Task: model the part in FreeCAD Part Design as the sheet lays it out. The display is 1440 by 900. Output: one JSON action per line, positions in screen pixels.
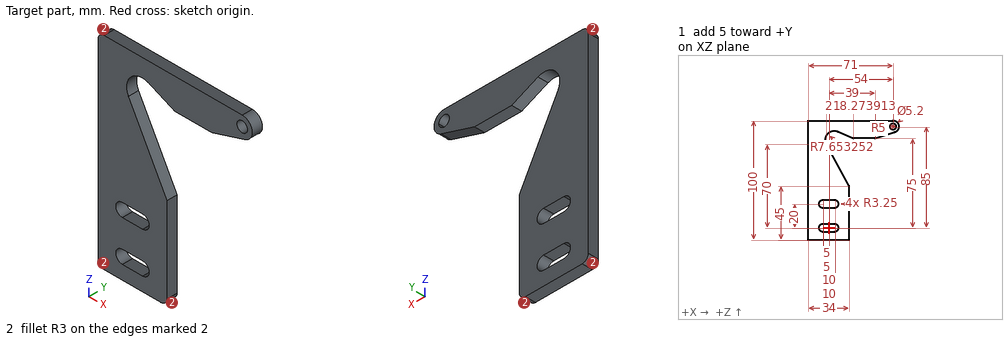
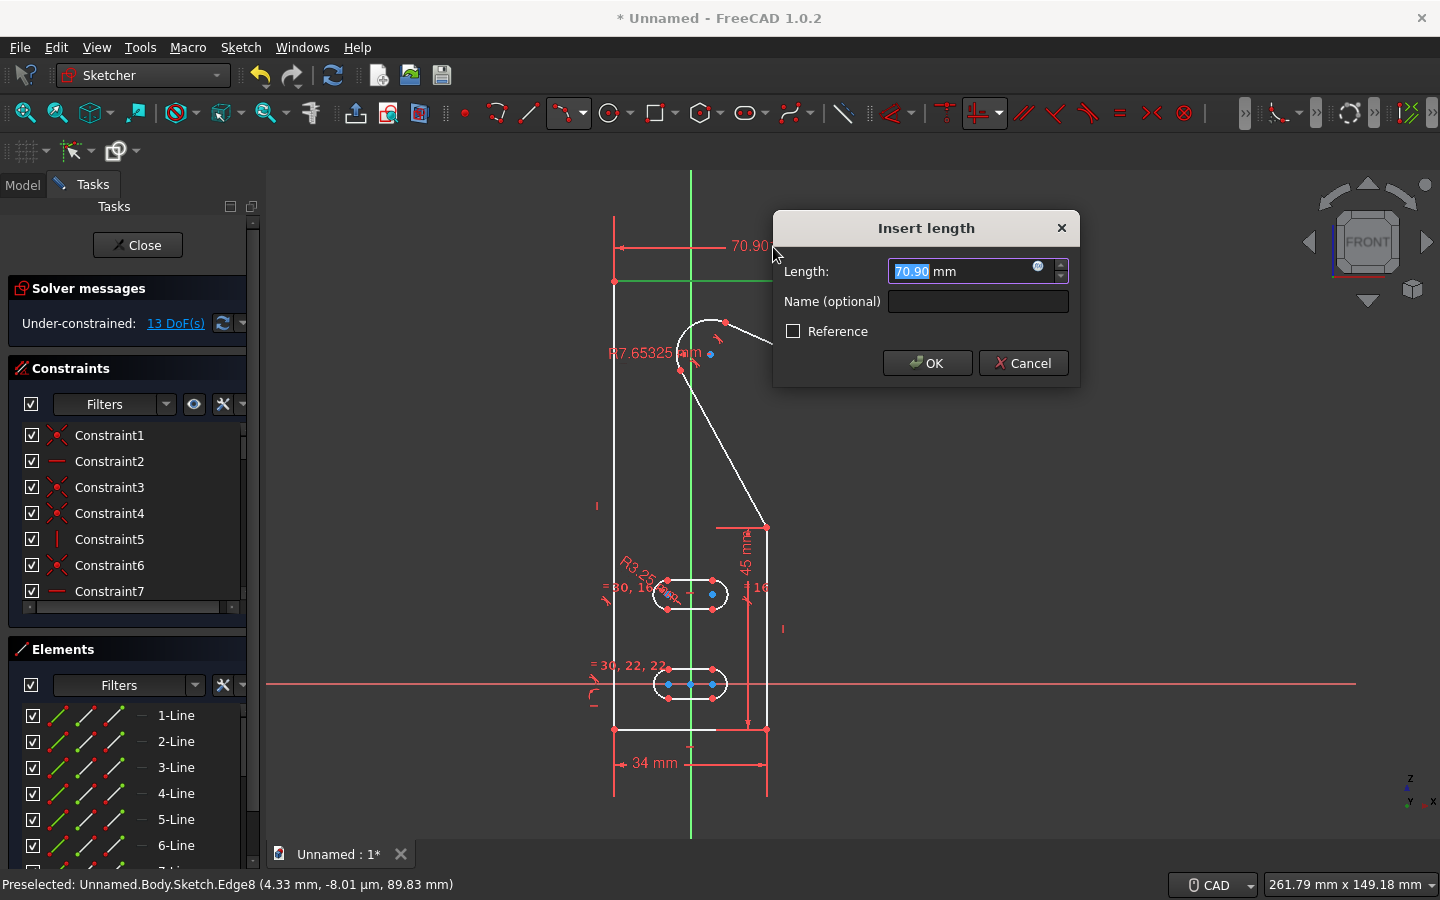
{"action": "type", "text": "71"}
{"action": "key", "text": "Return"}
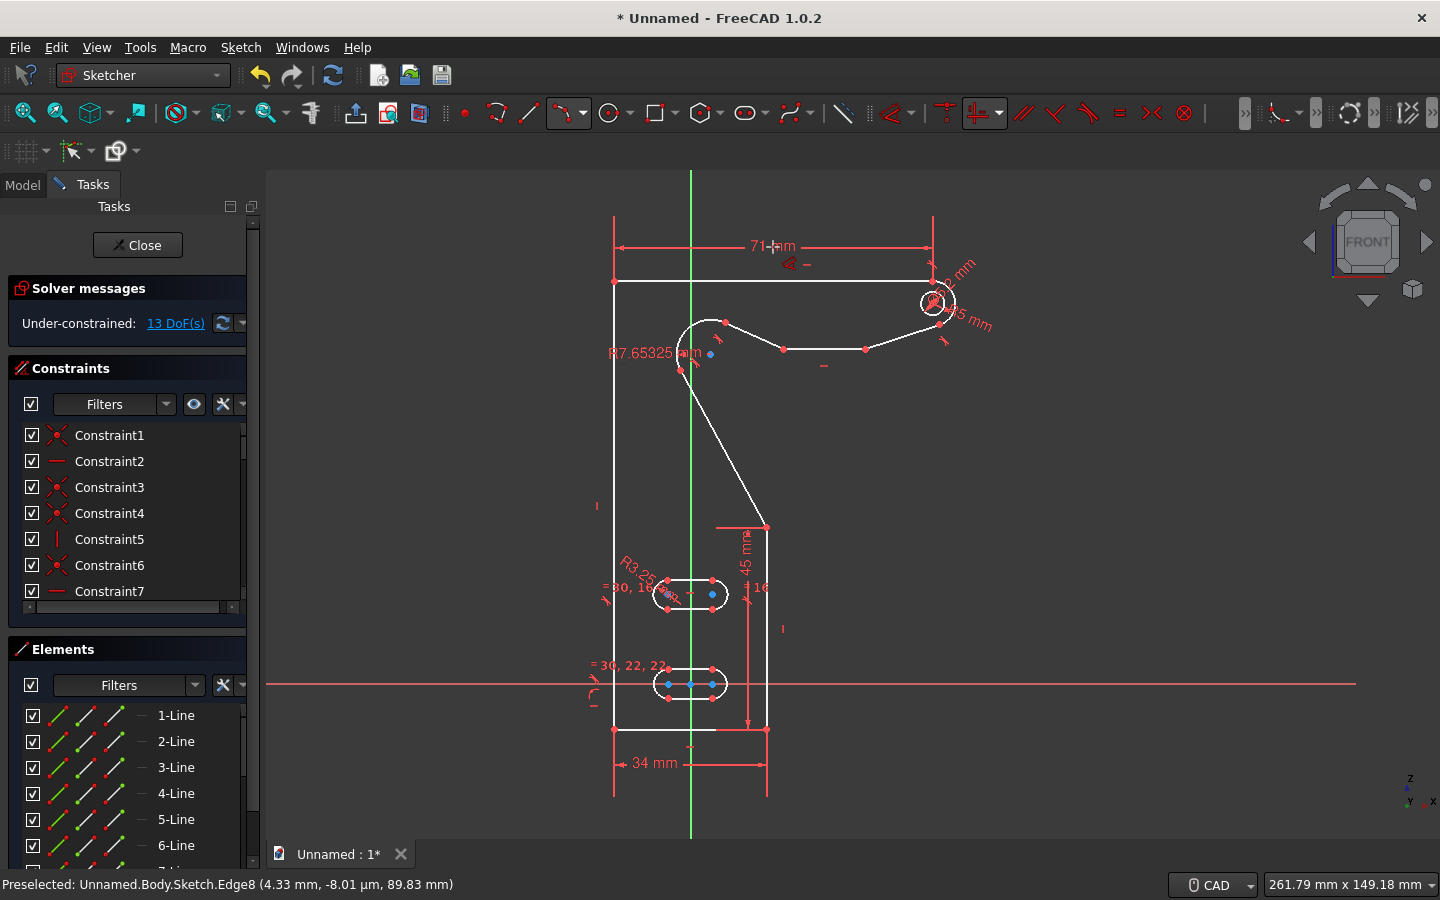
{"action": "scroll", "coordinate": [681, 580], "scroll_direction": "up", "scroll_amount": 3}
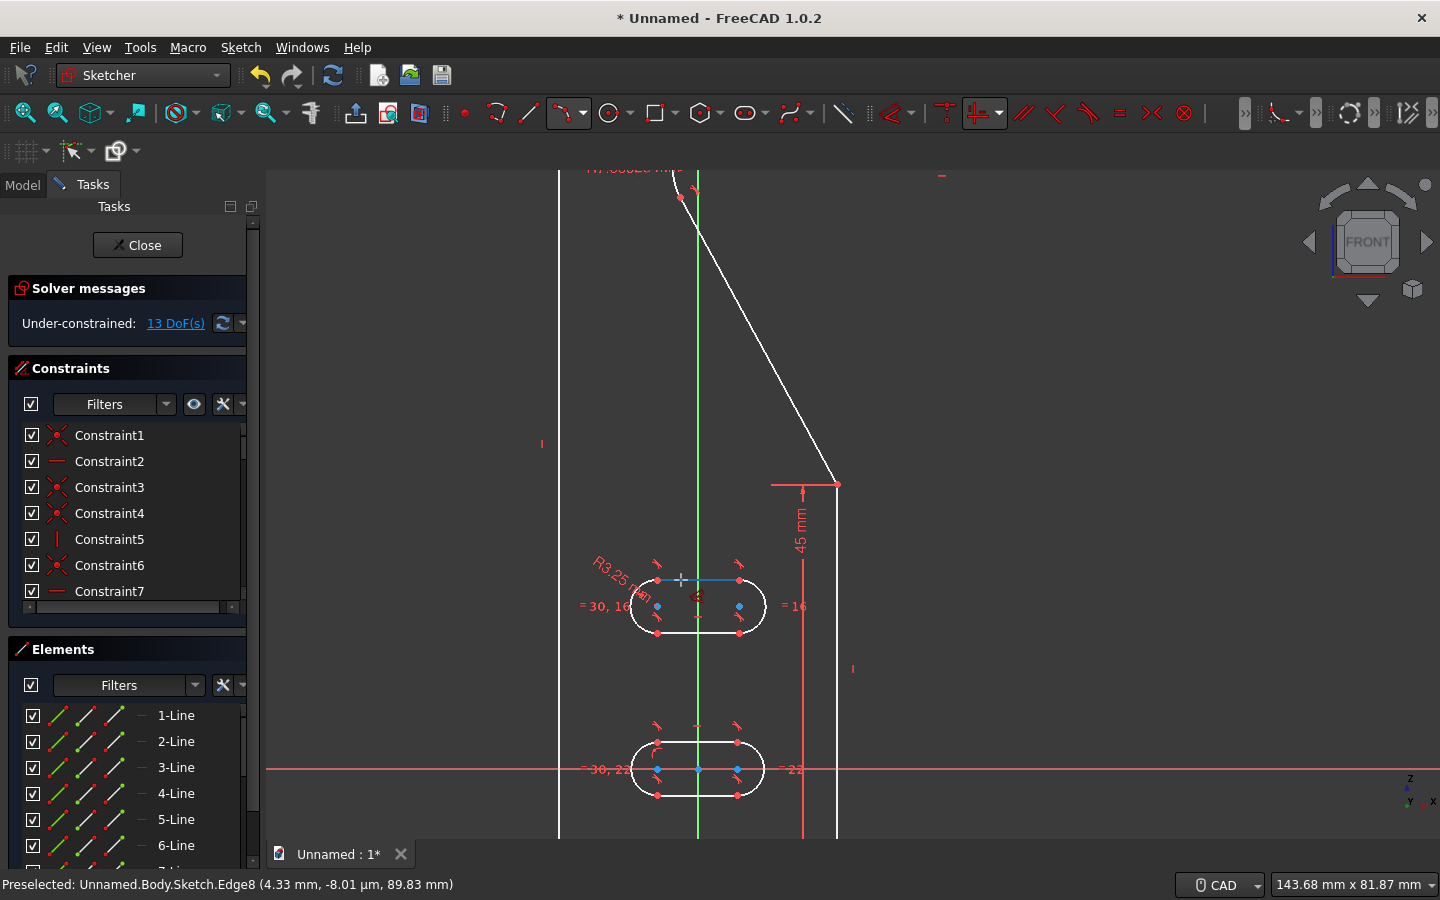
{"action": "left_click", "coordinate": [682, 580]}
{"action": "left_click", "coordinate": [679, 614]}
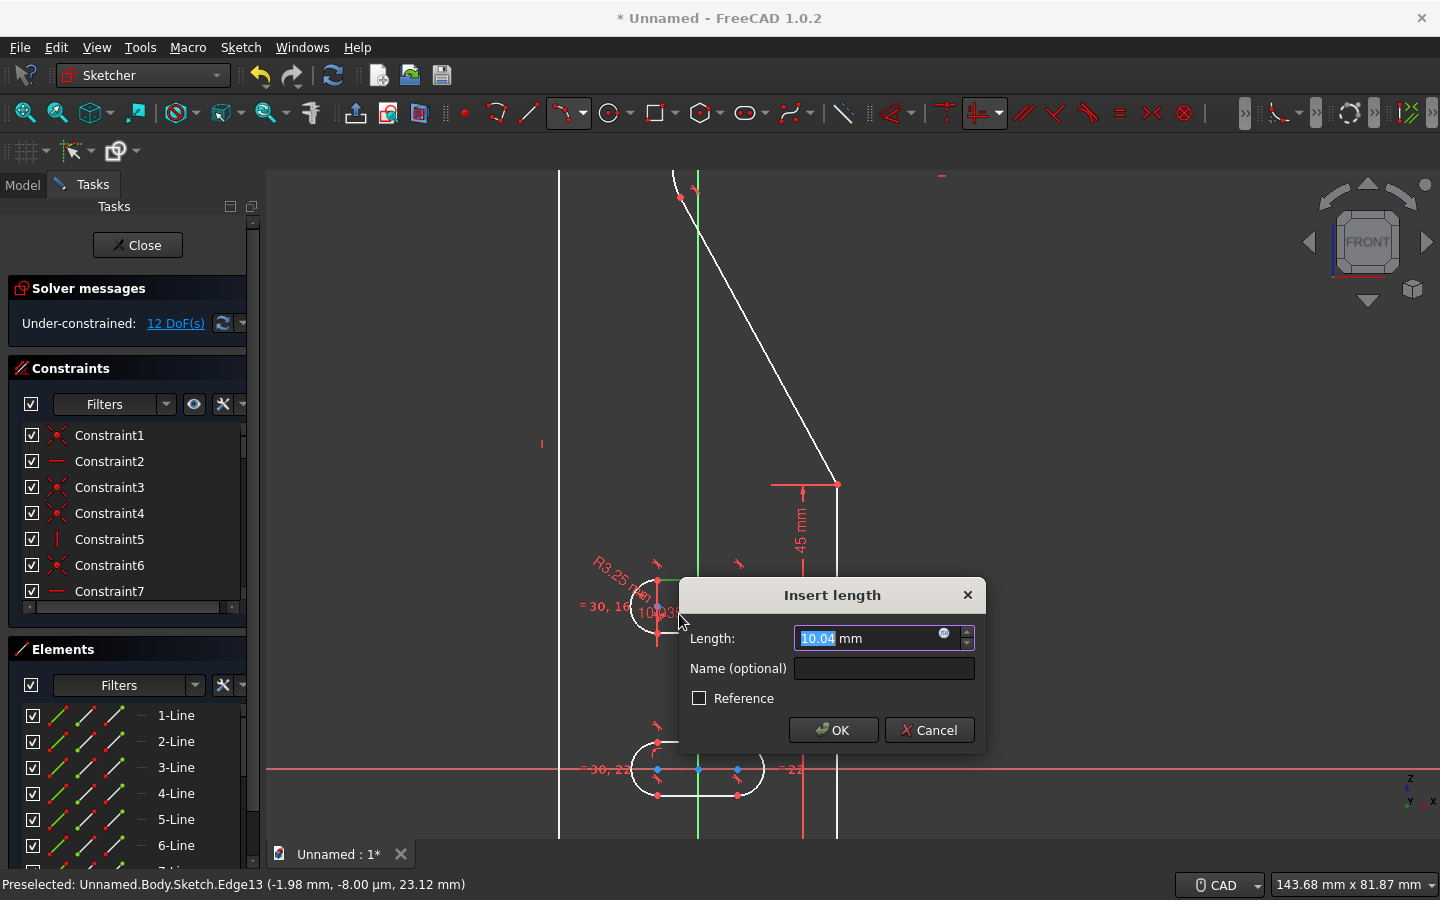
{"action": "type", "text": "10"}
{"action": "key", "text": "Return"}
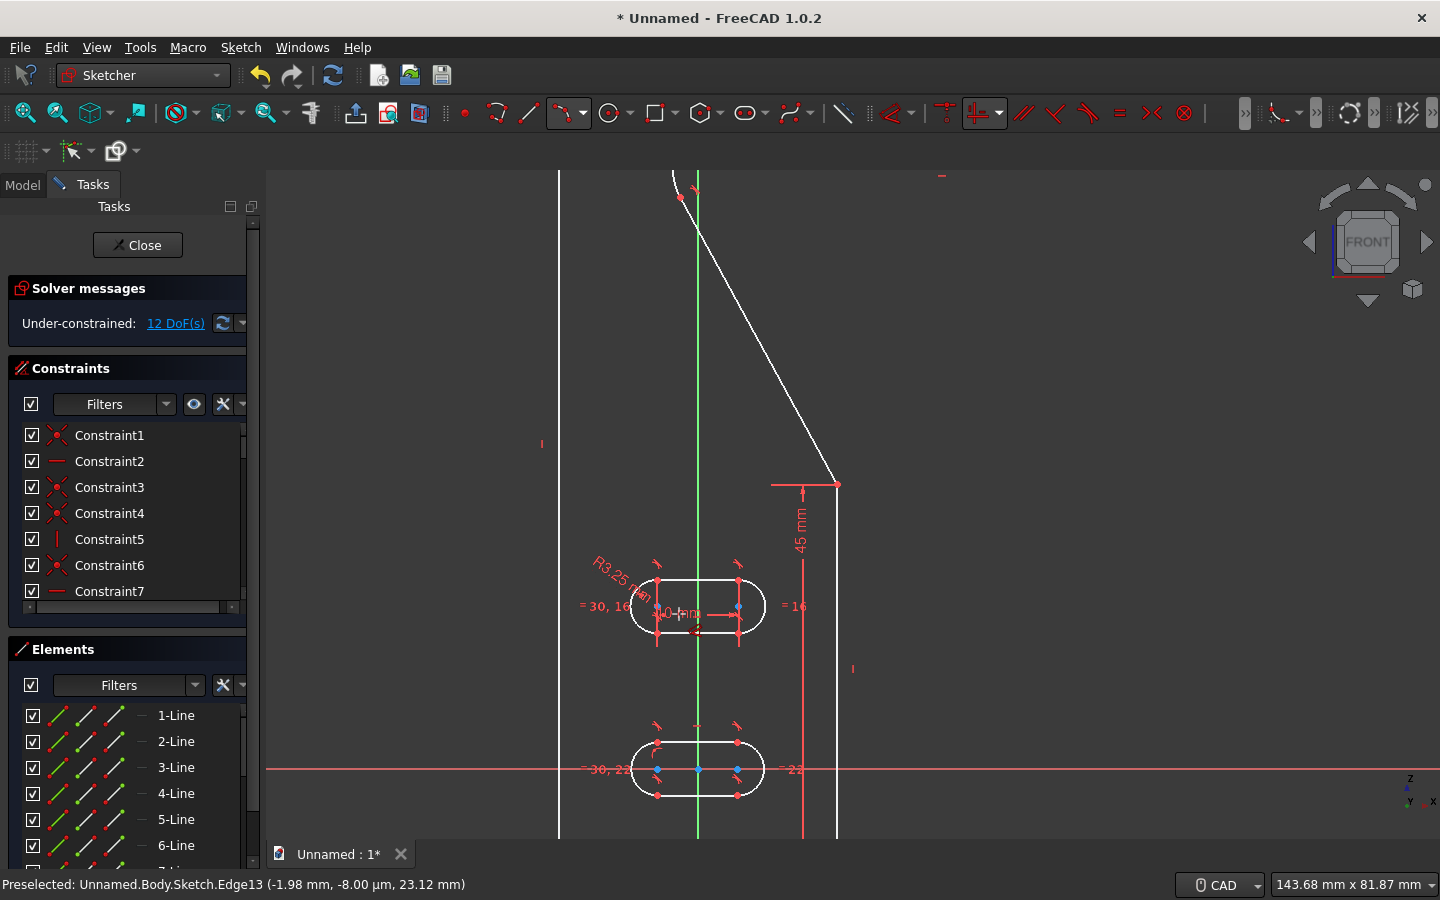
{"action": "left_click", "coordinate": [682, 742]}
{"action": "left_click", "coordinate": [679, 708]}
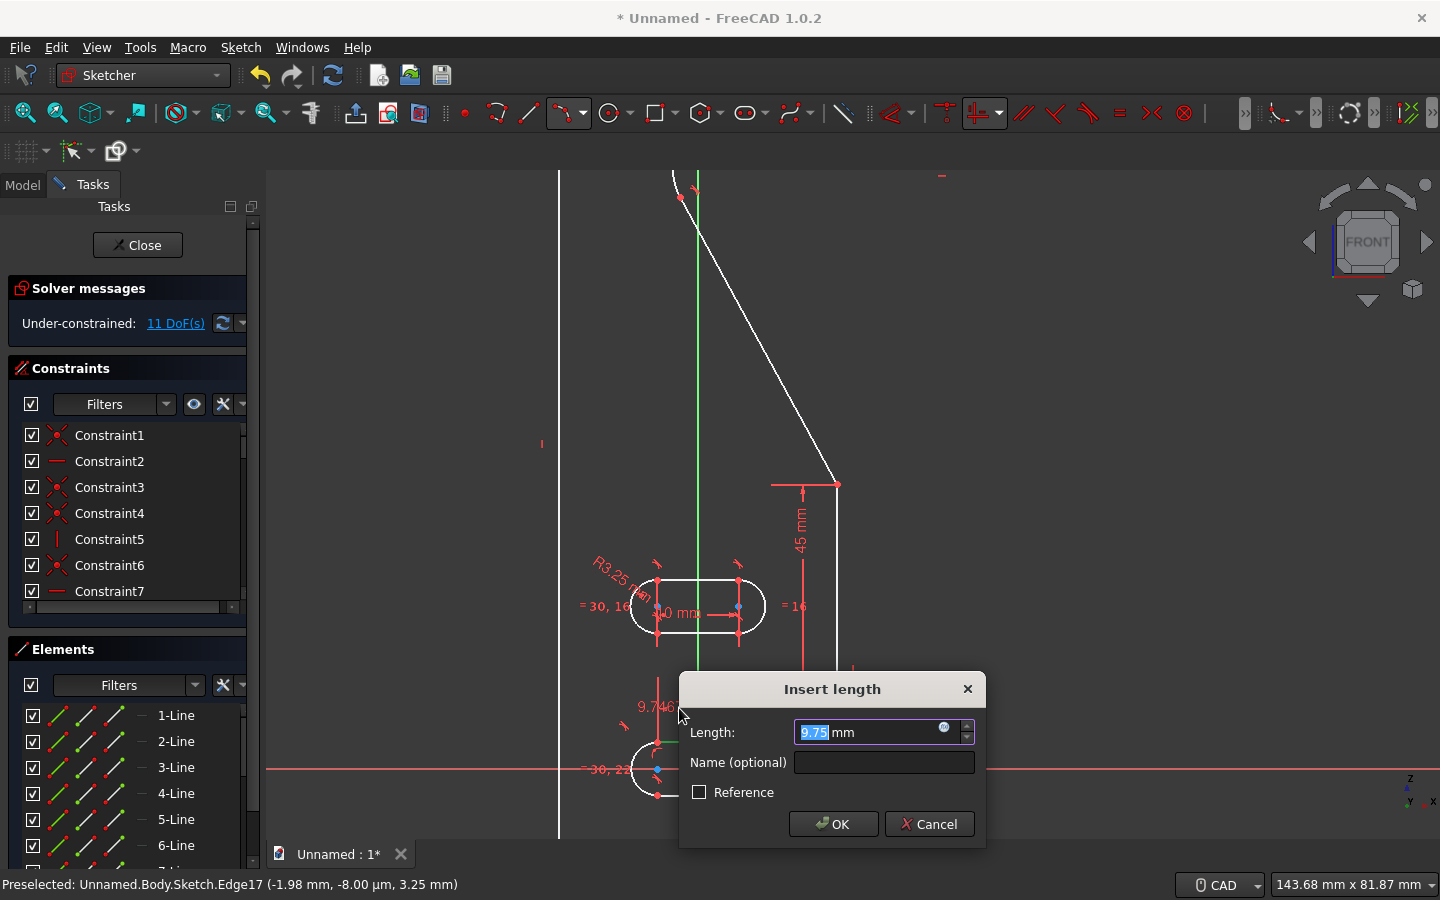
{"action": "type", "text": "10"}
{"action": "key", "text": "Return"}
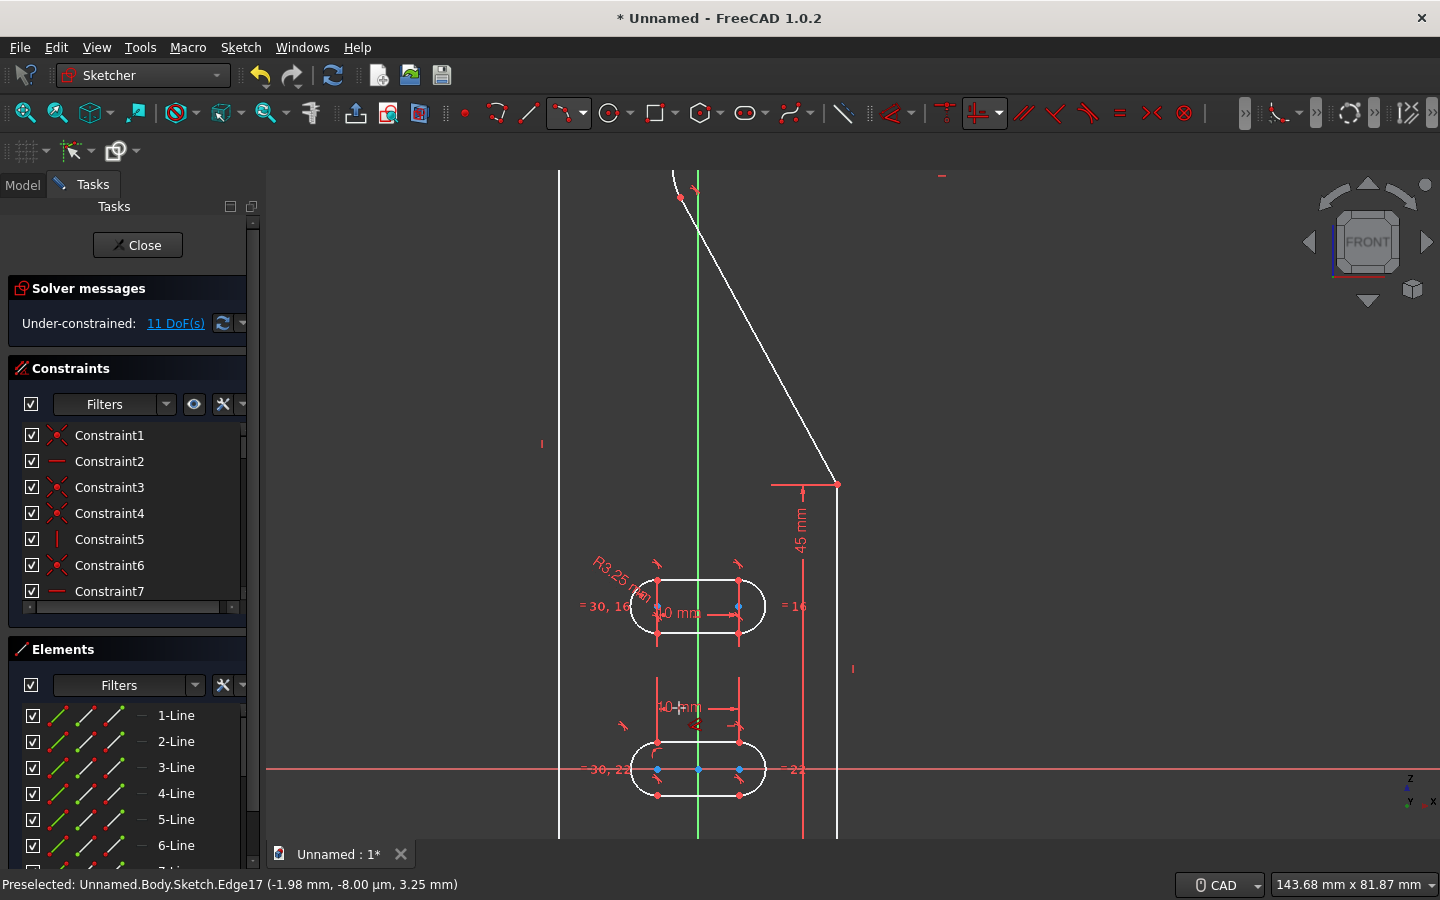
{"action": "scroll", "coordinate": [681, 580], "scroll_direction": "down", "scroll_amount": 3}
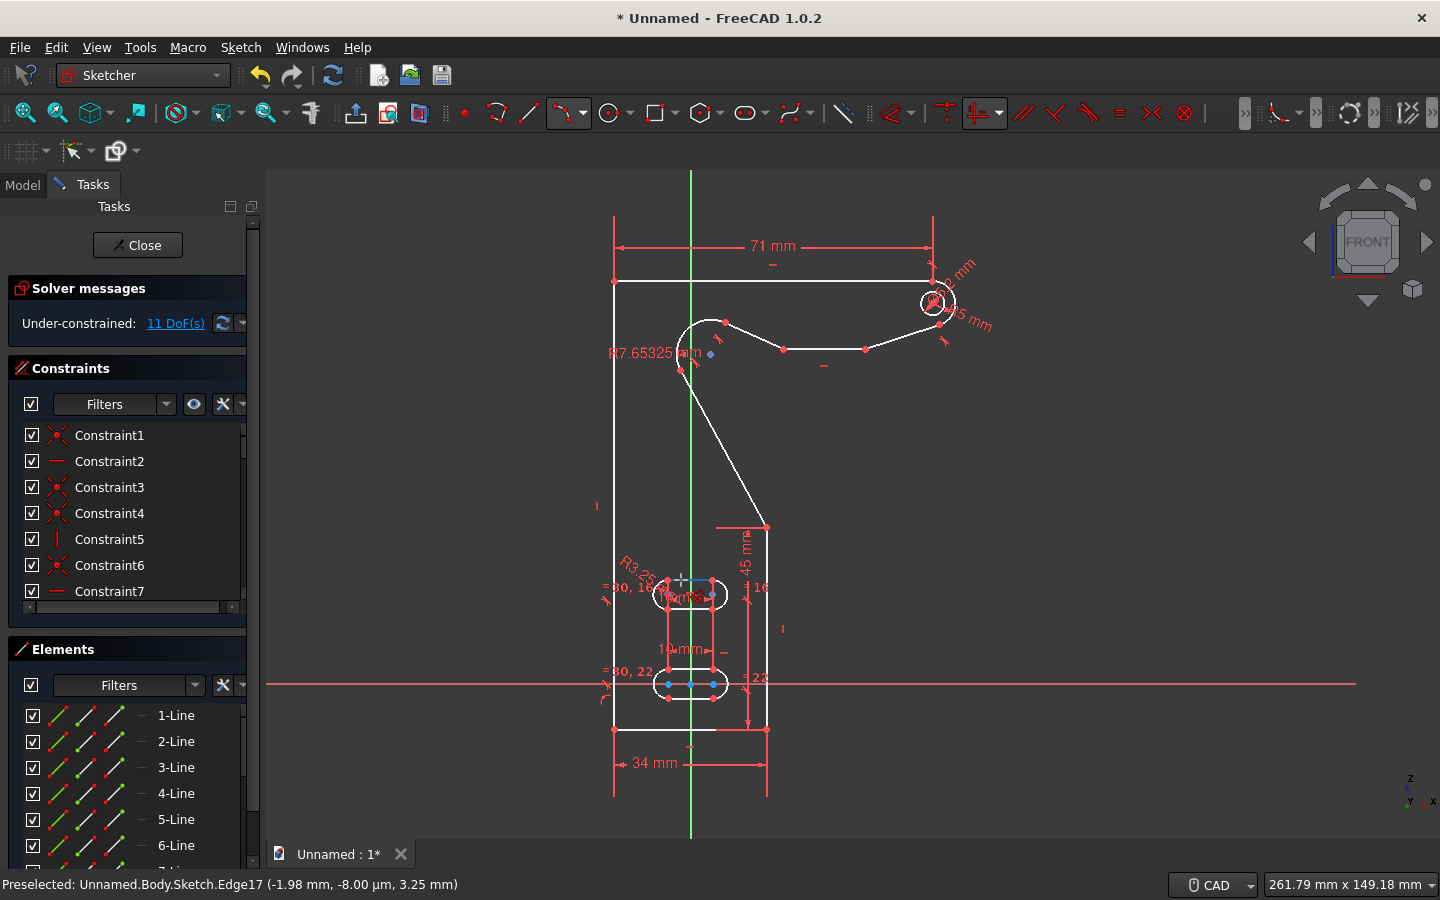
{"action": "scroll", "coordinate": [681, 371], "scroll_direction": "up", "scroll_amount": 8}